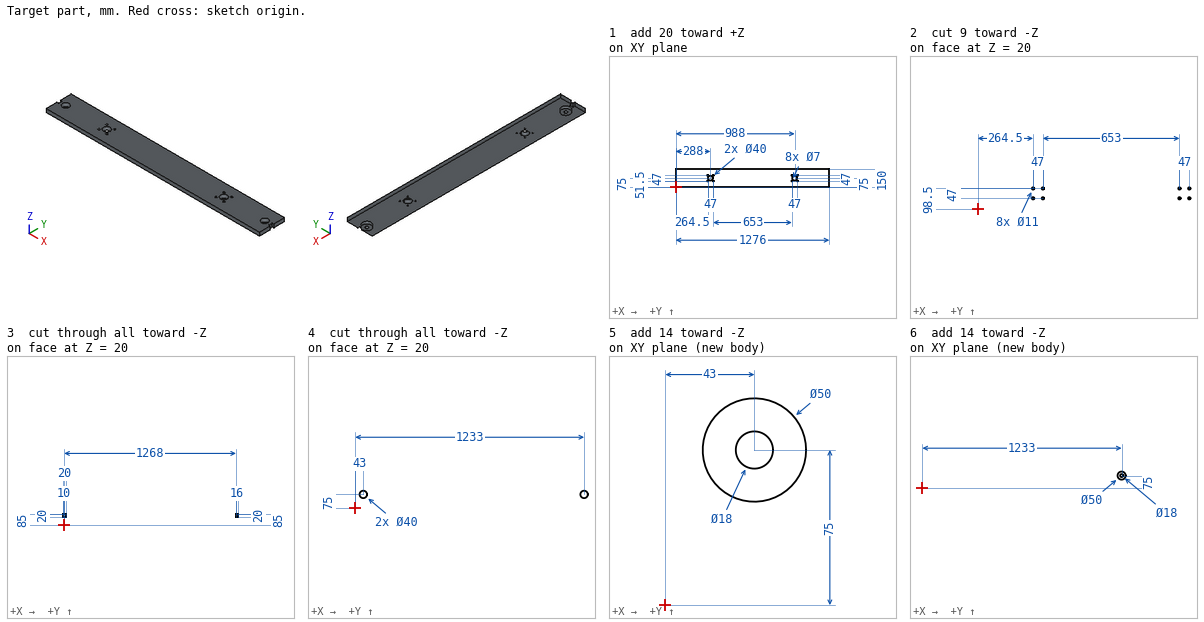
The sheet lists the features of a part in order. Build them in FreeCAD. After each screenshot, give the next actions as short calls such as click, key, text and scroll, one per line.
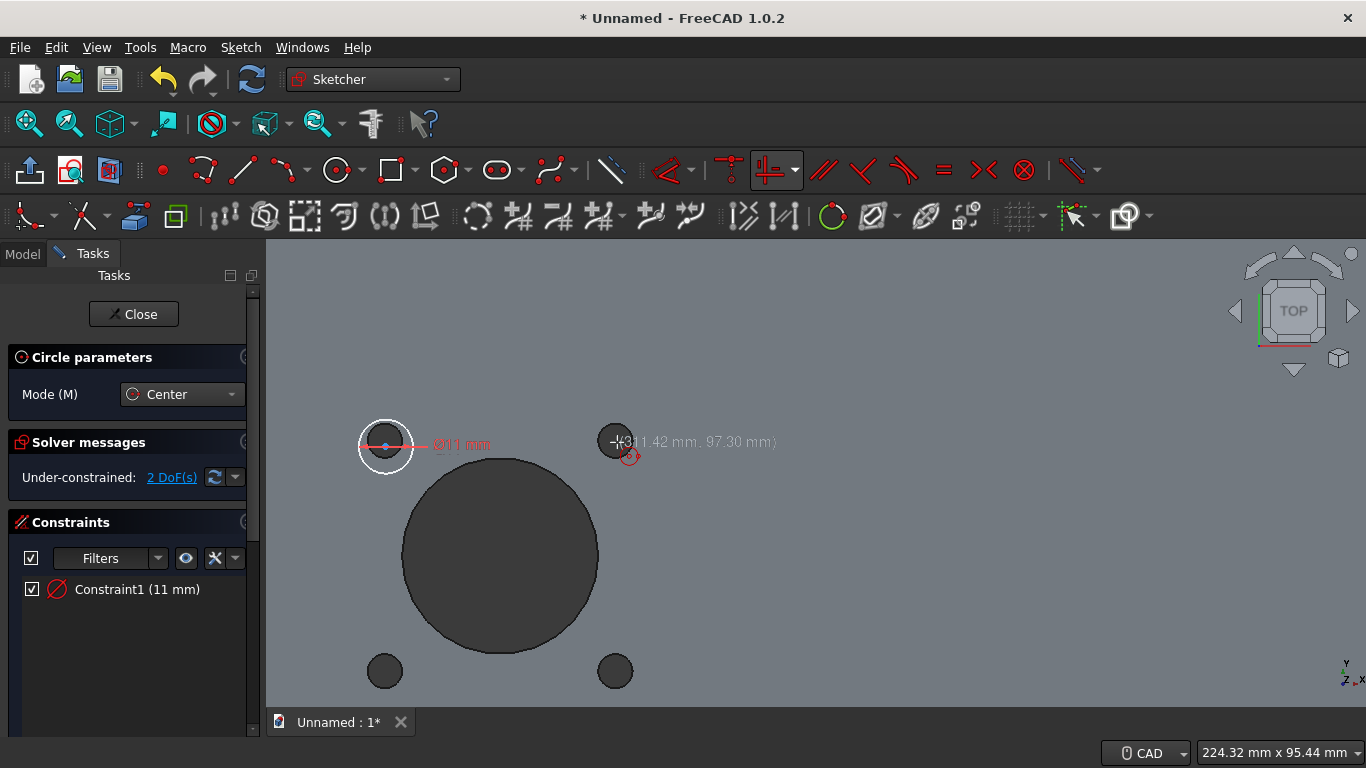
scroll(617, 442, down, 10)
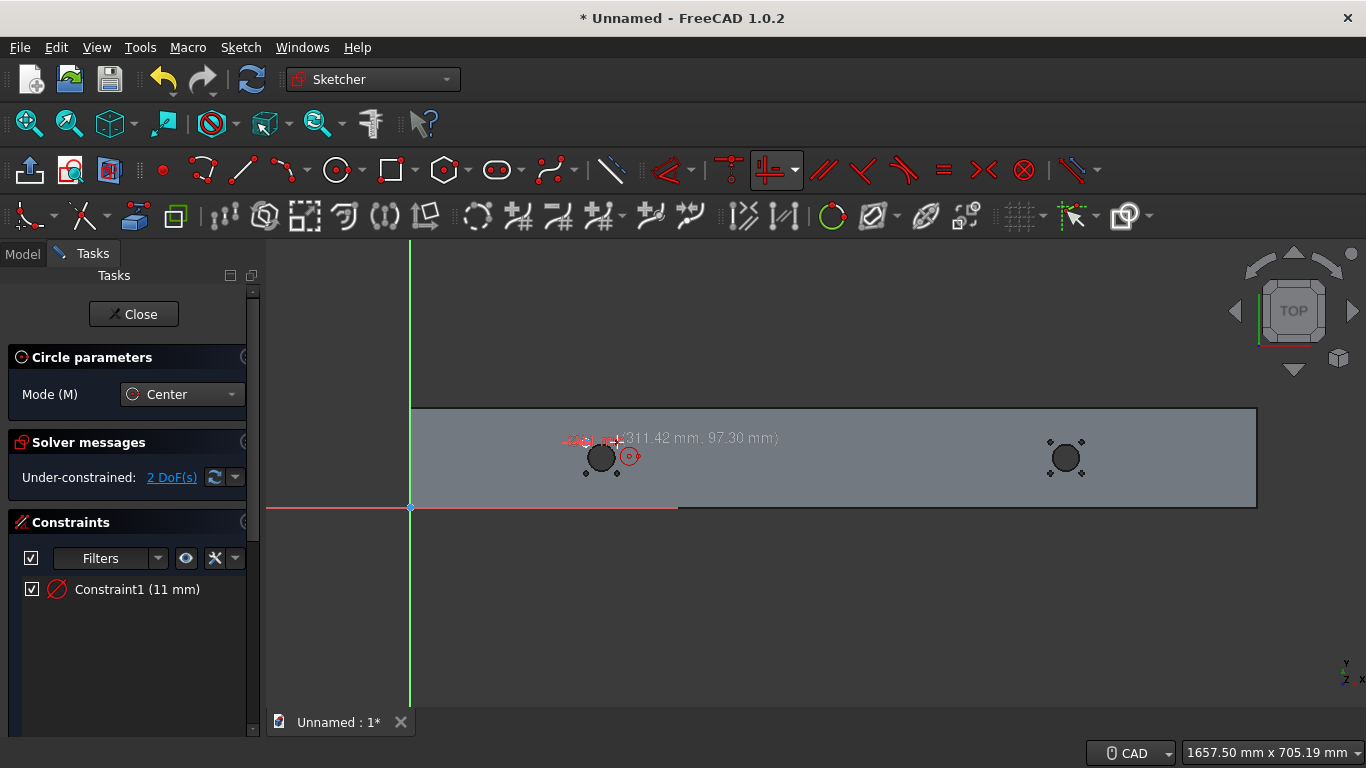
click(617, 442)
move(620, 440)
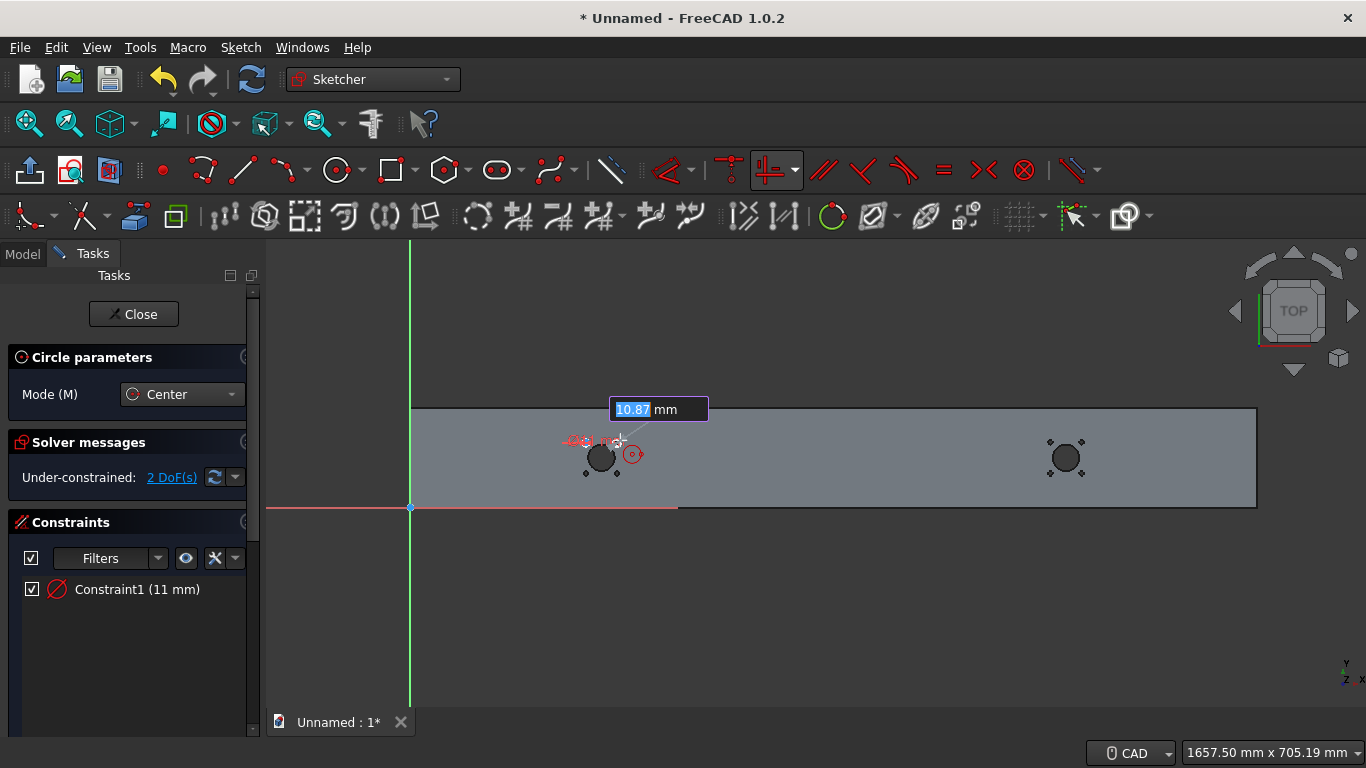
text(11)
key(Return)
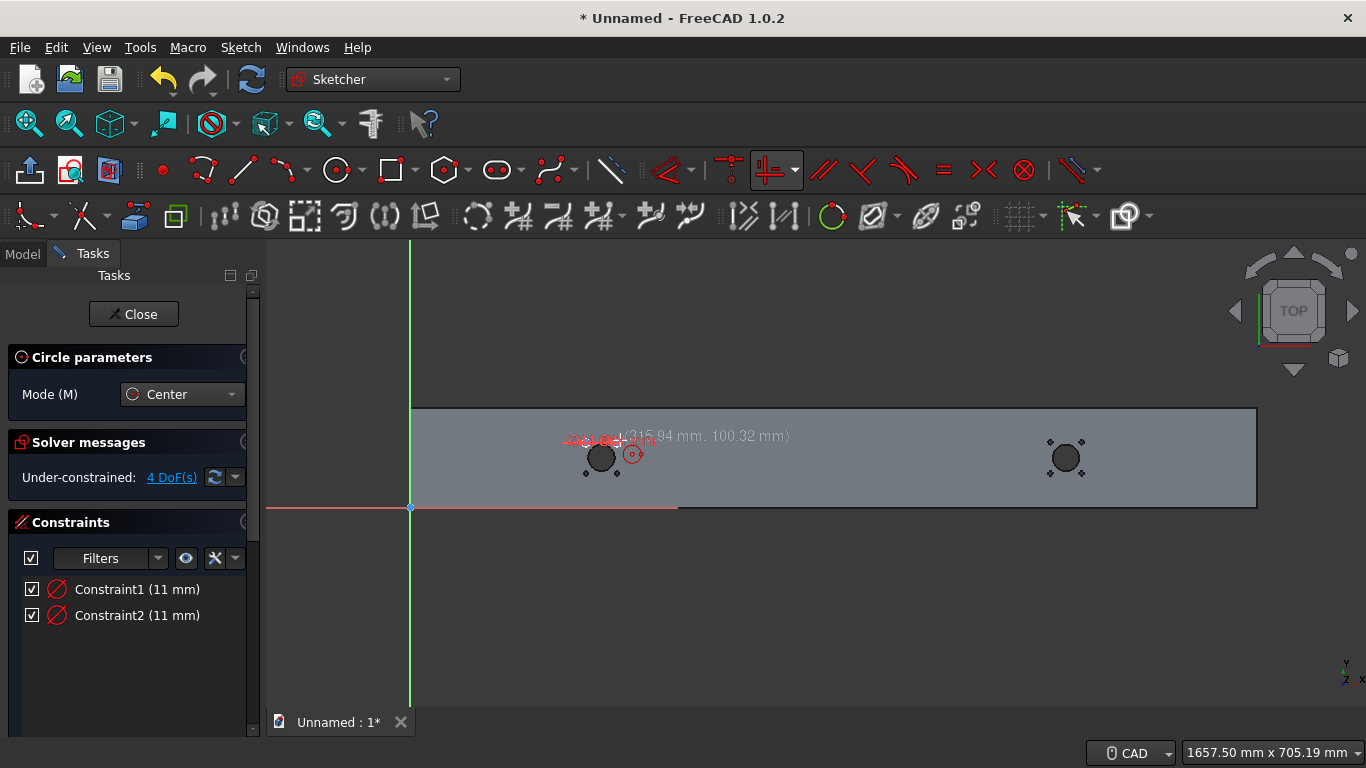
scroll(617, 473, up, 10)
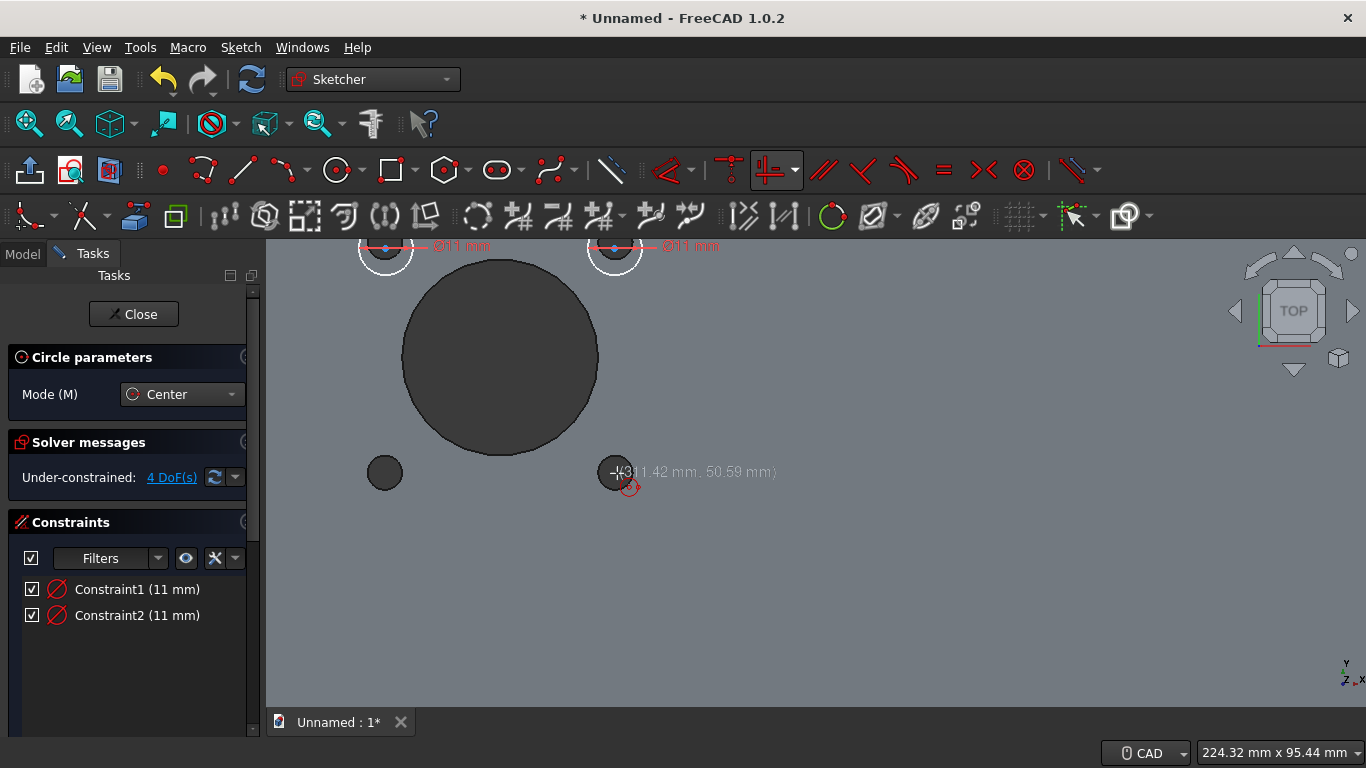
scroll(617, 473, down, 10)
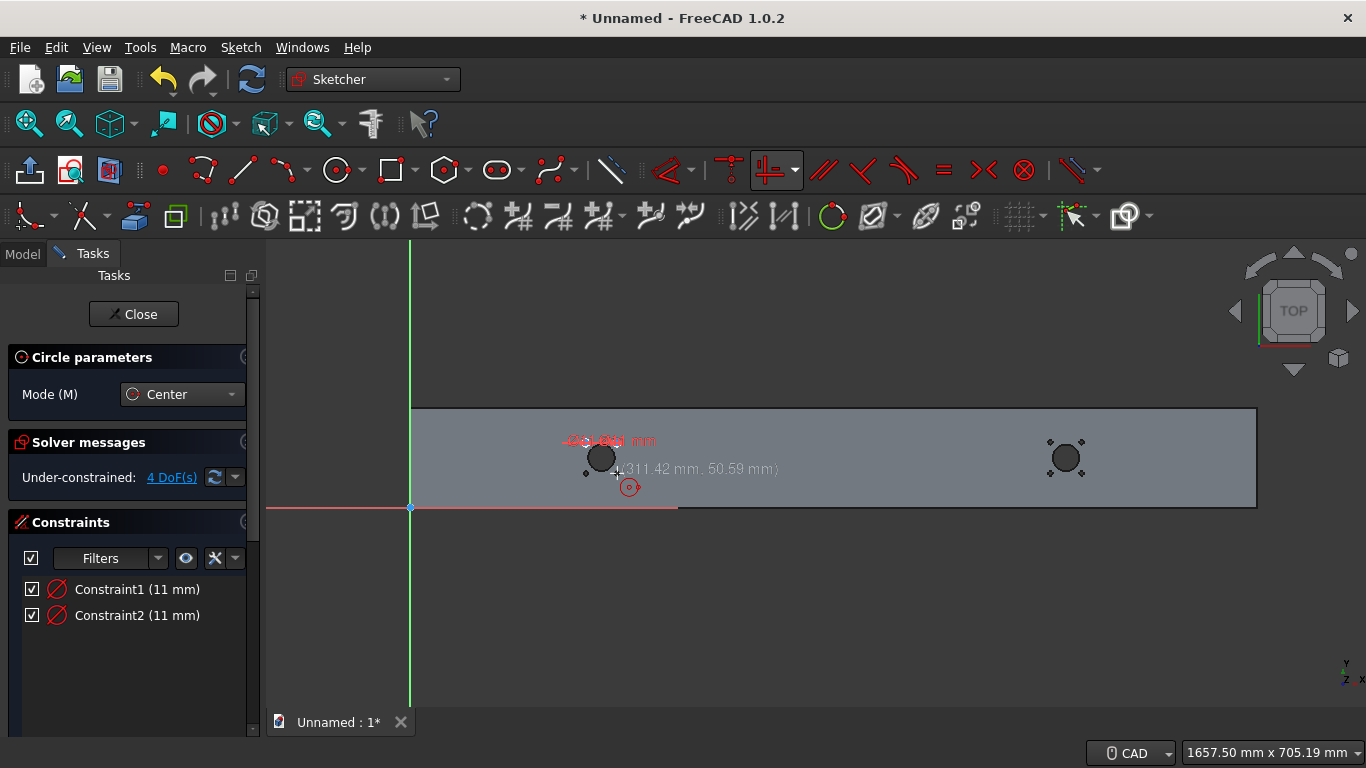
click(617, 473)
move(620, 471)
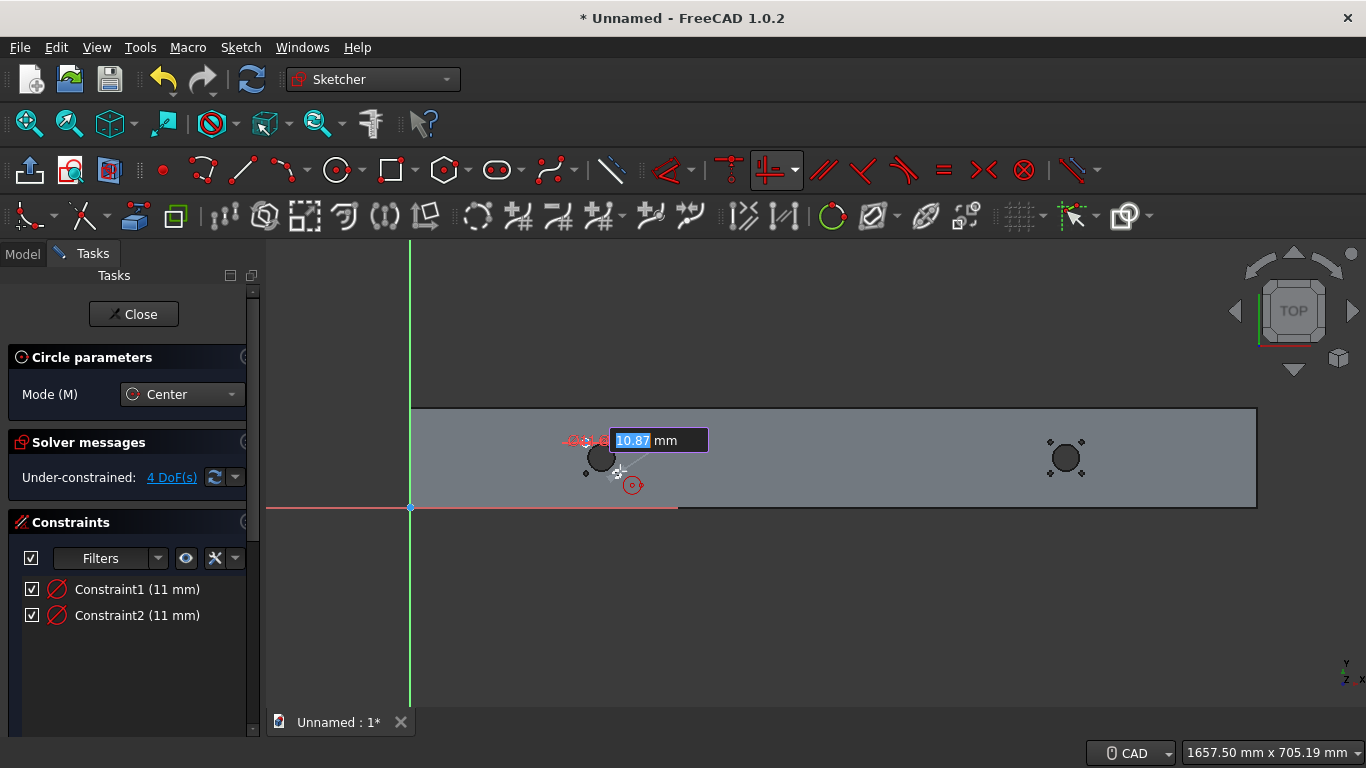
text(11)
key(Return)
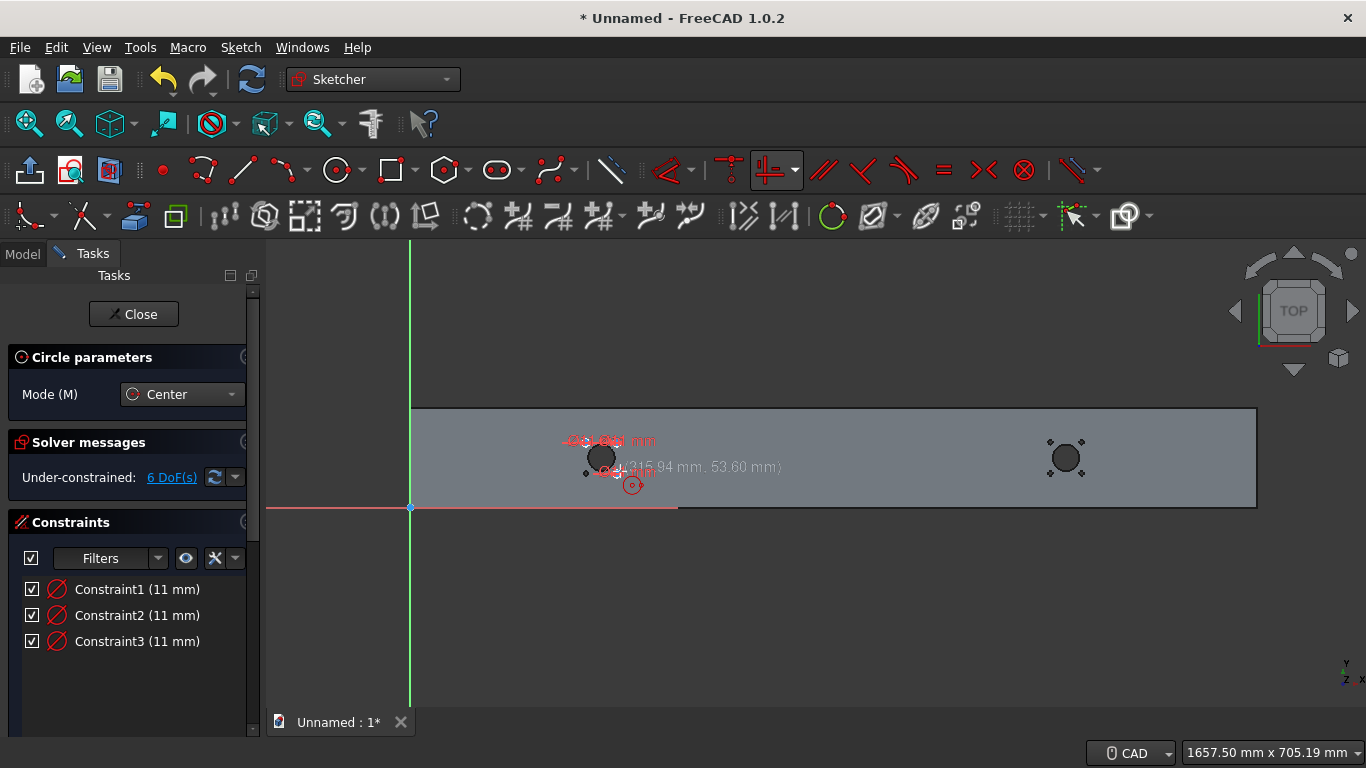
scroll(586, 473, up, 10)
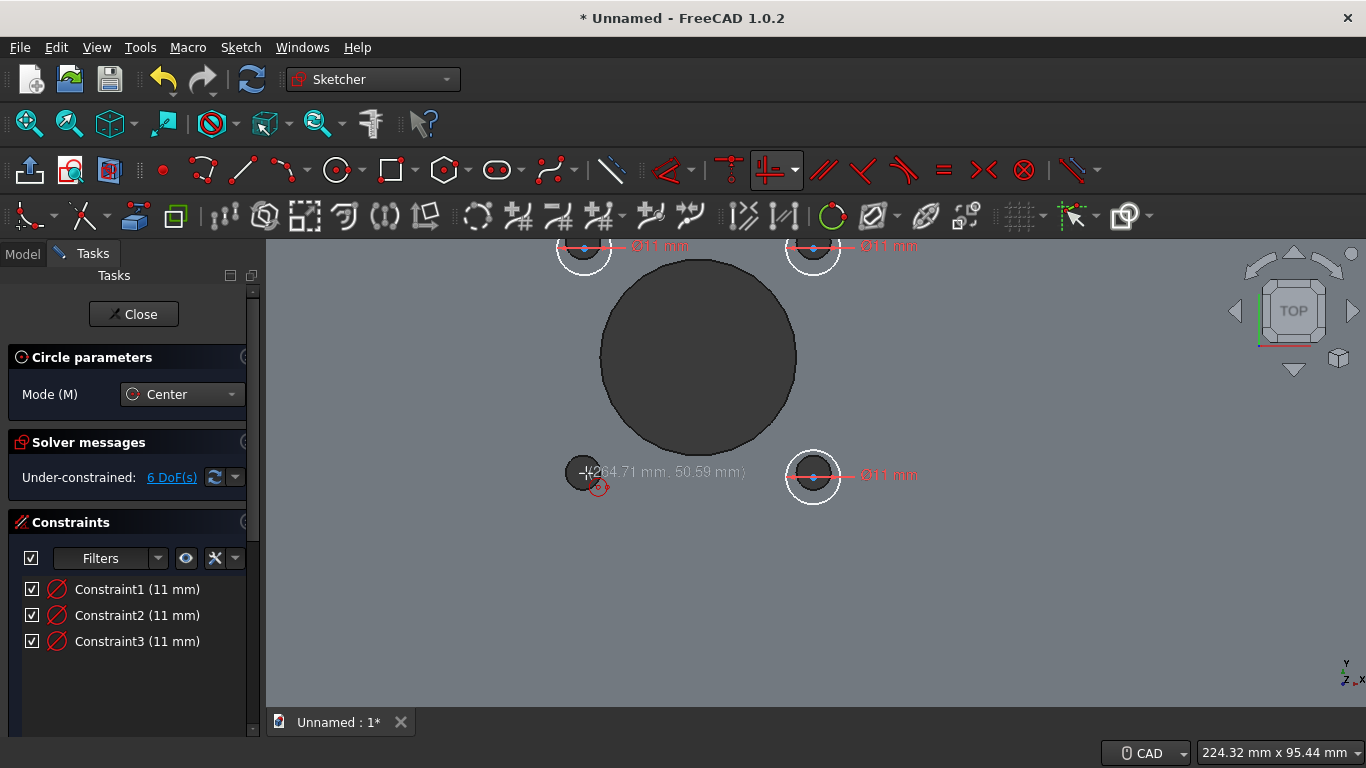
scroll(586, 473, down, 10)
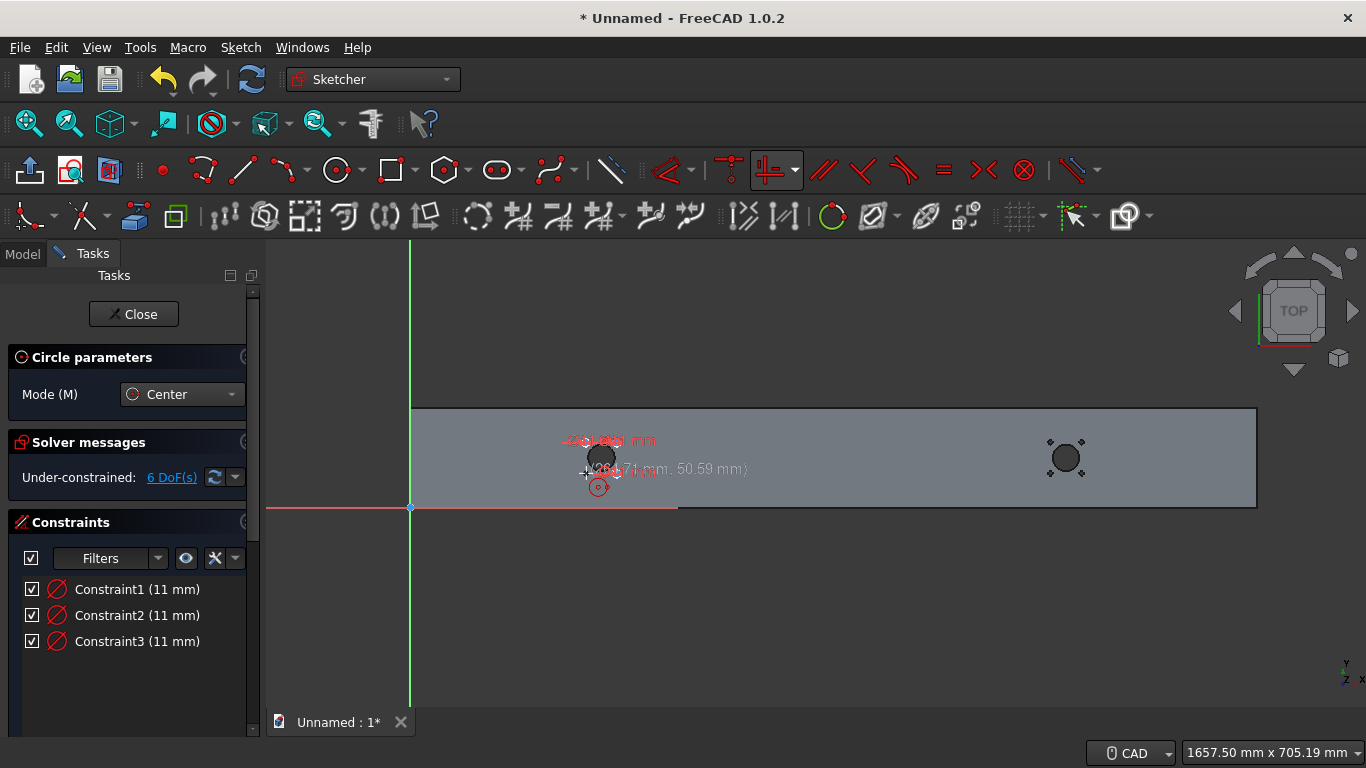
click(586, 473)
move(588, 471)